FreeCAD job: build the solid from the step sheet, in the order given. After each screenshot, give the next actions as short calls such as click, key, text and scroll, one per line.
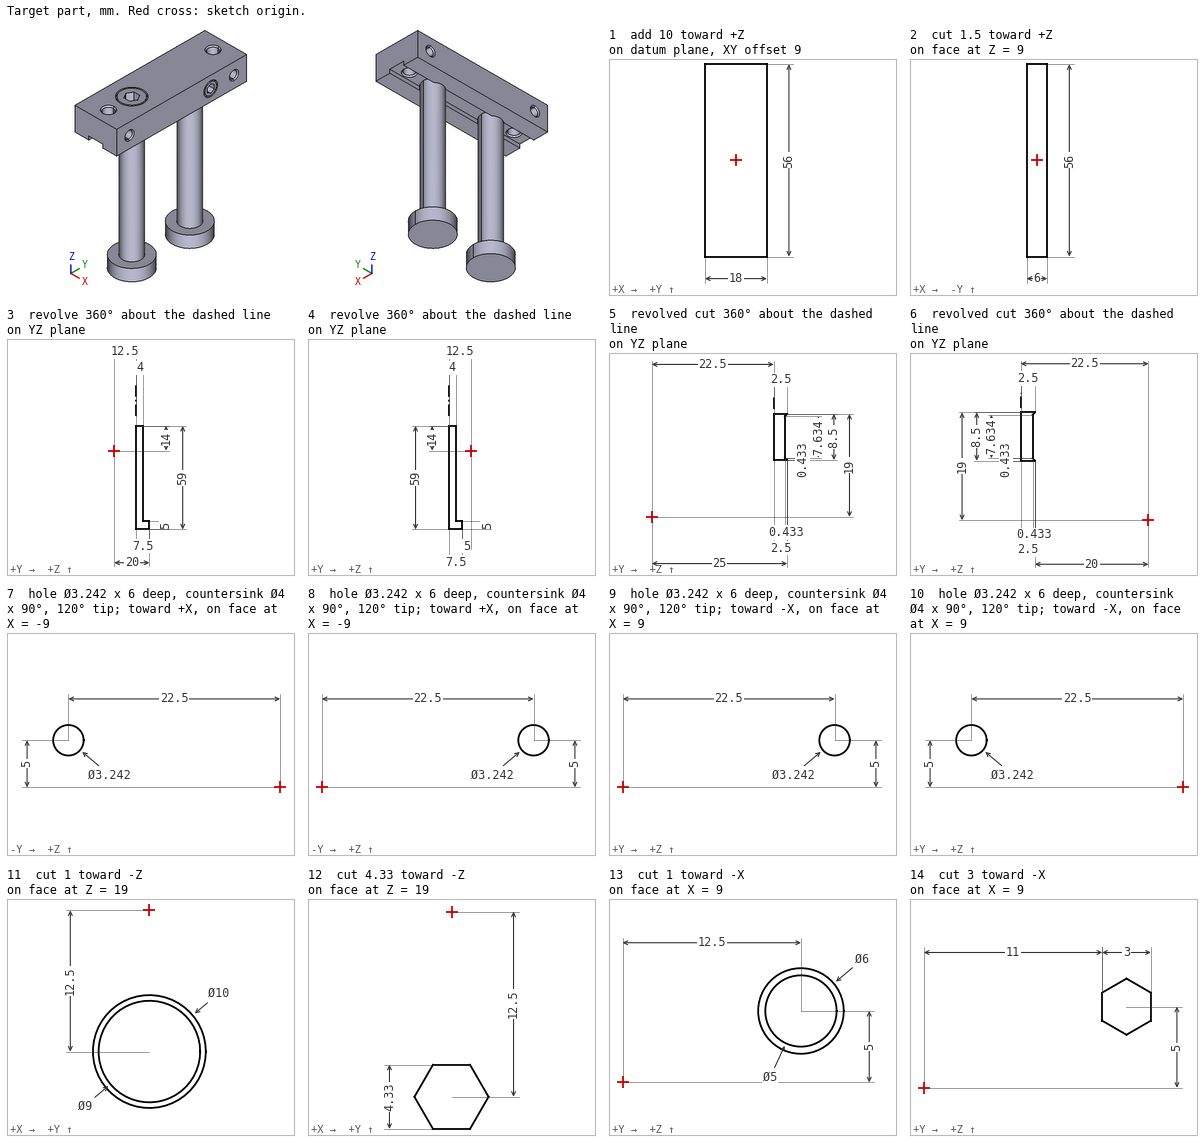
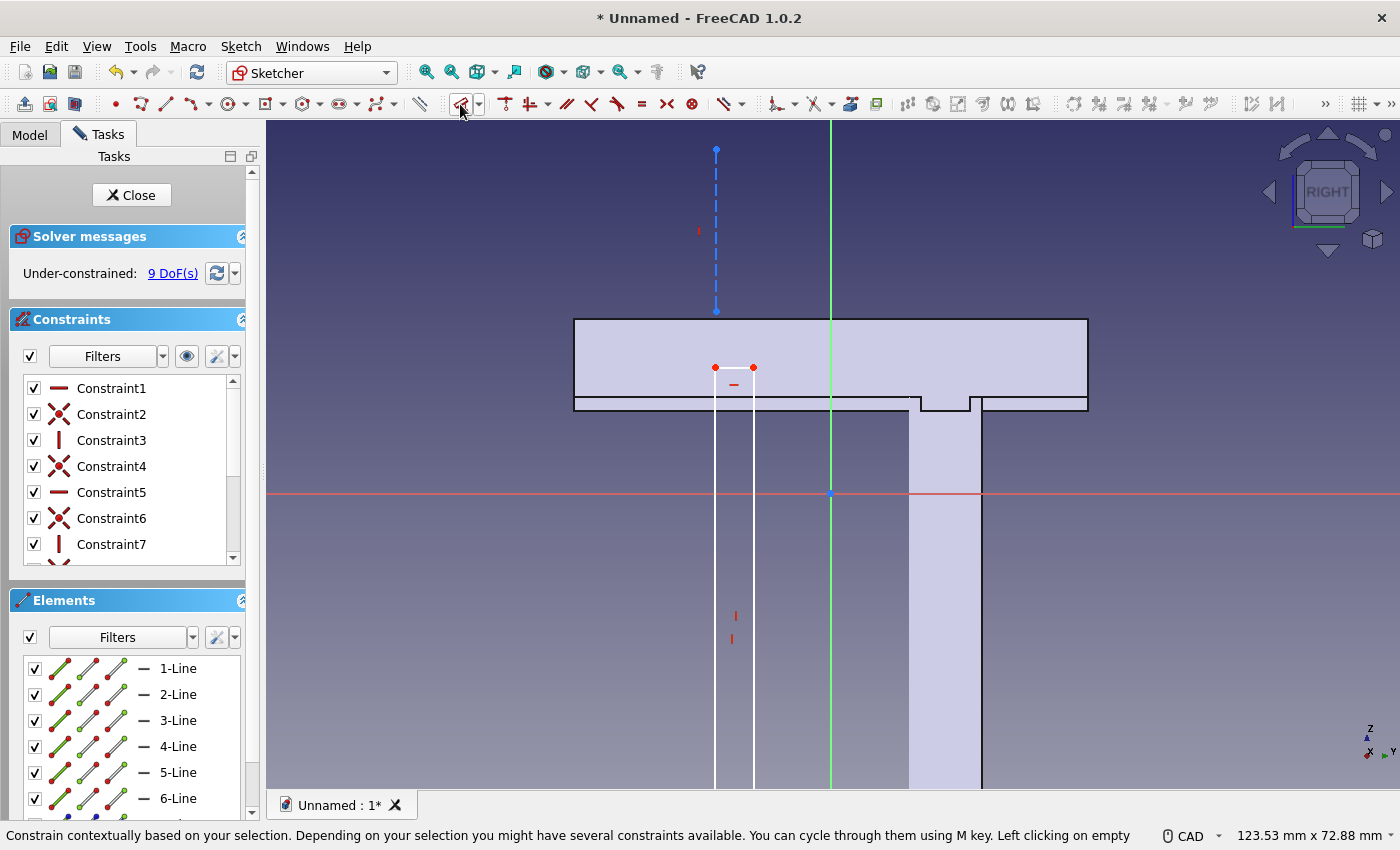
click(742, 368)
click(735, 334)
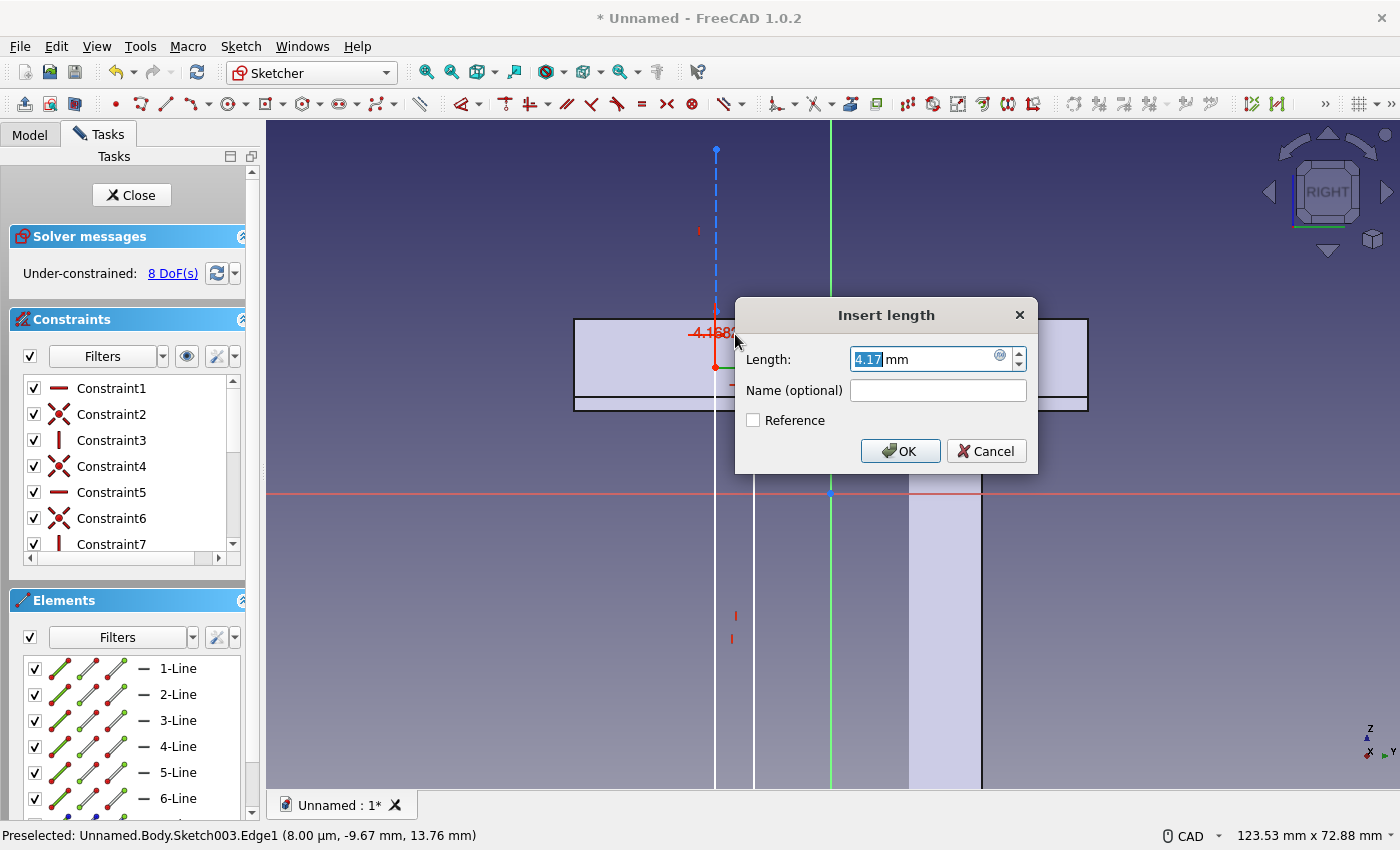
text(4)
key(Return)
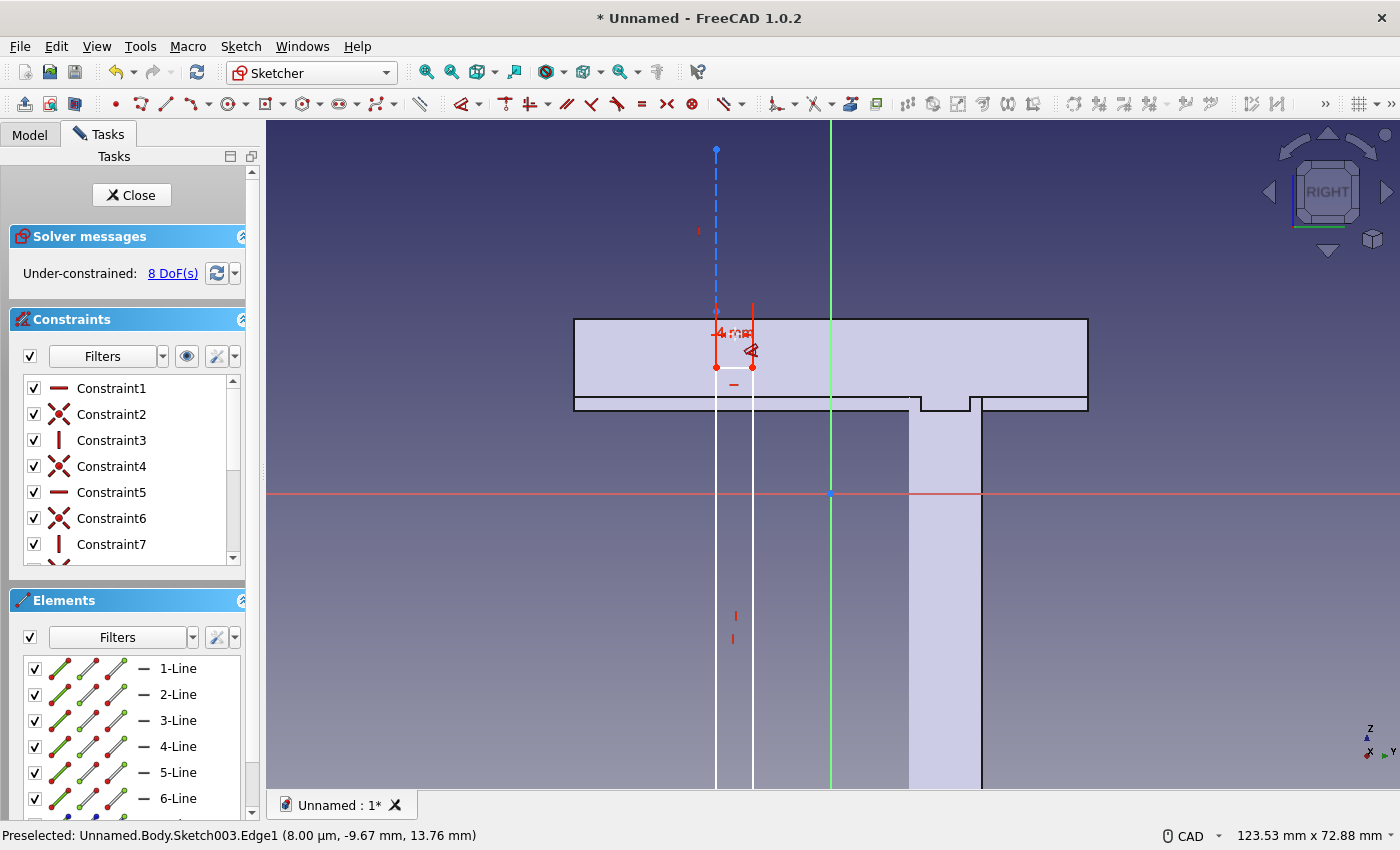
scroll(754, 365, down, 3)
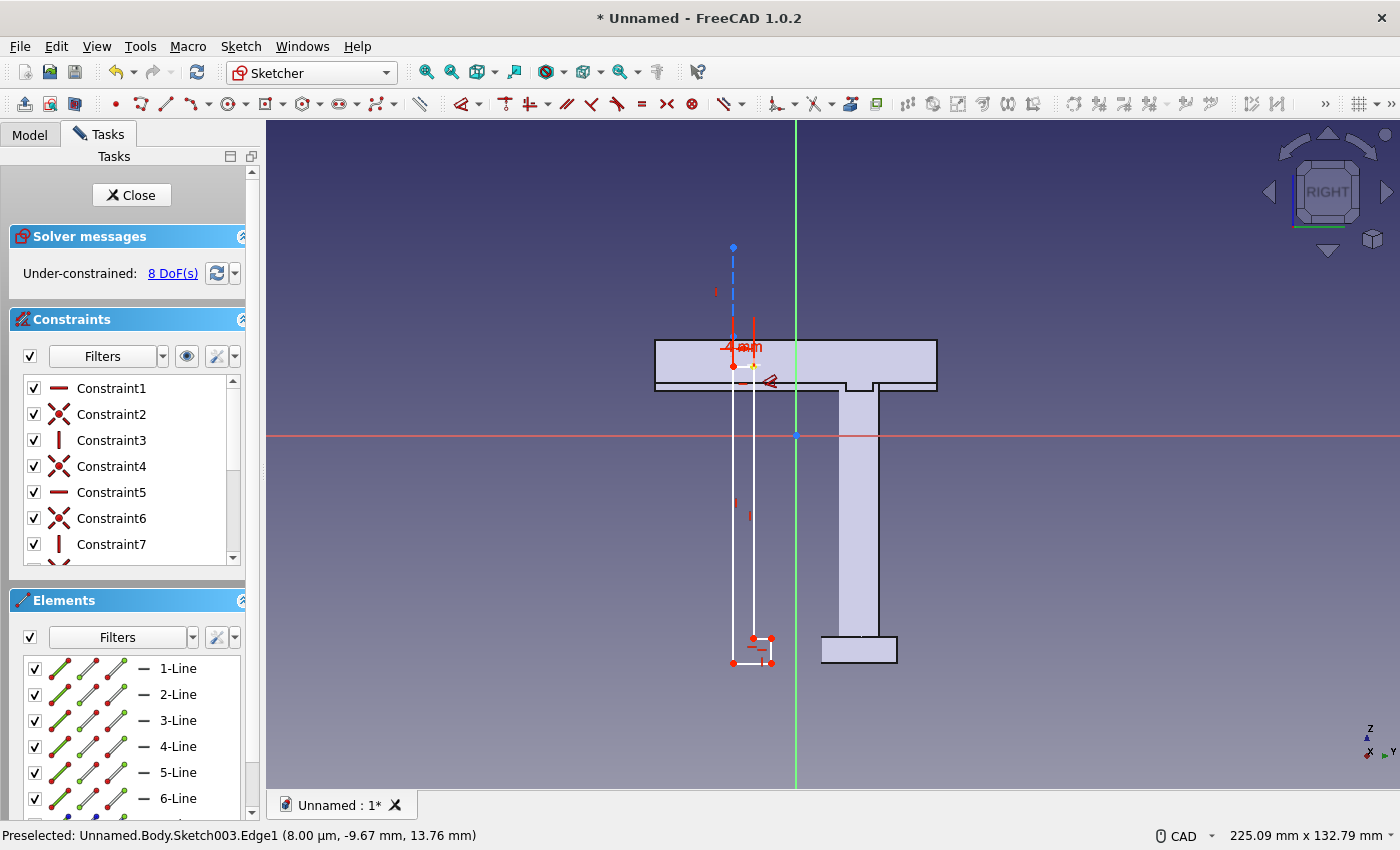
scroll(771, 656, up, 4)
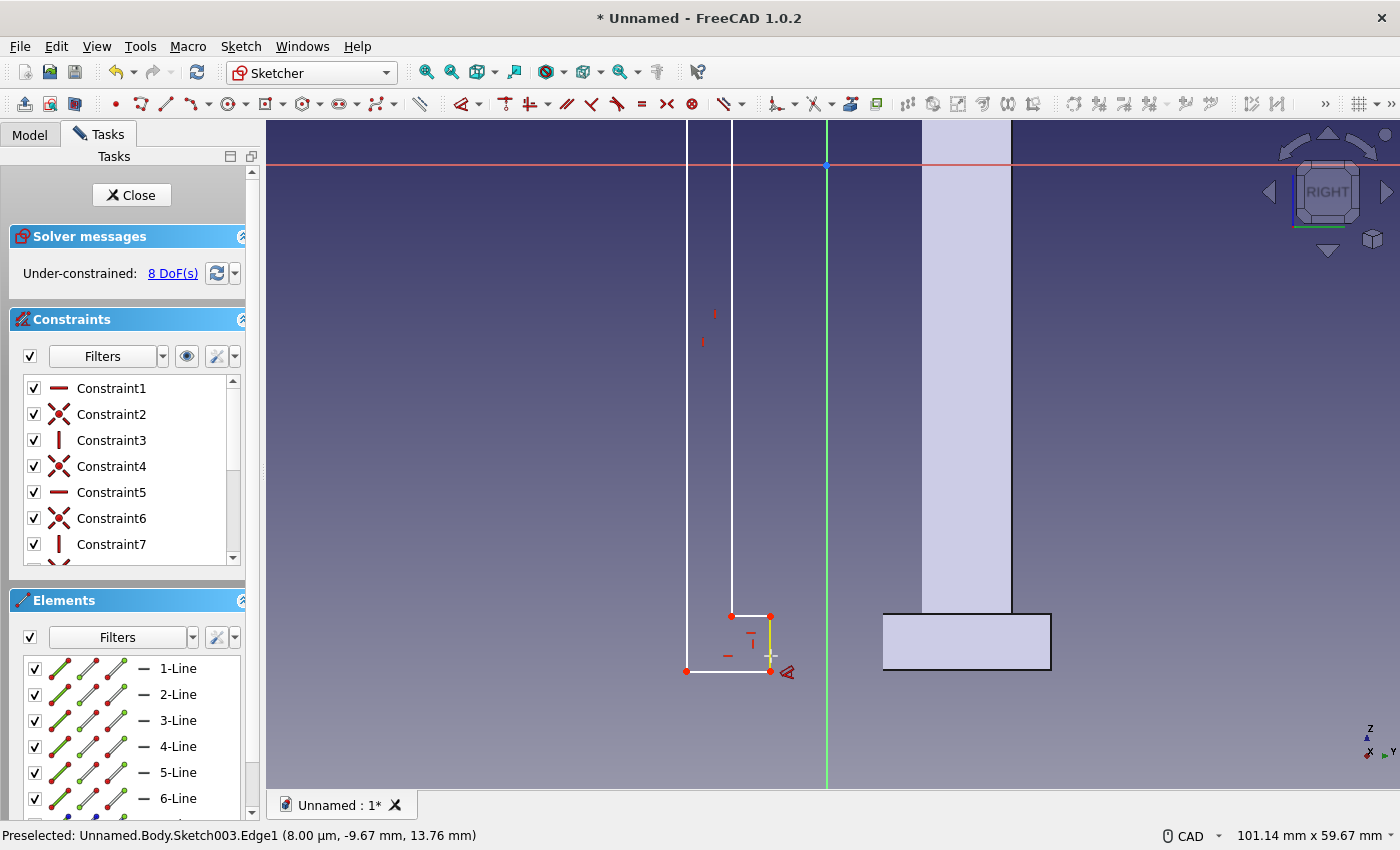
click(770, 655)
click(804, 644)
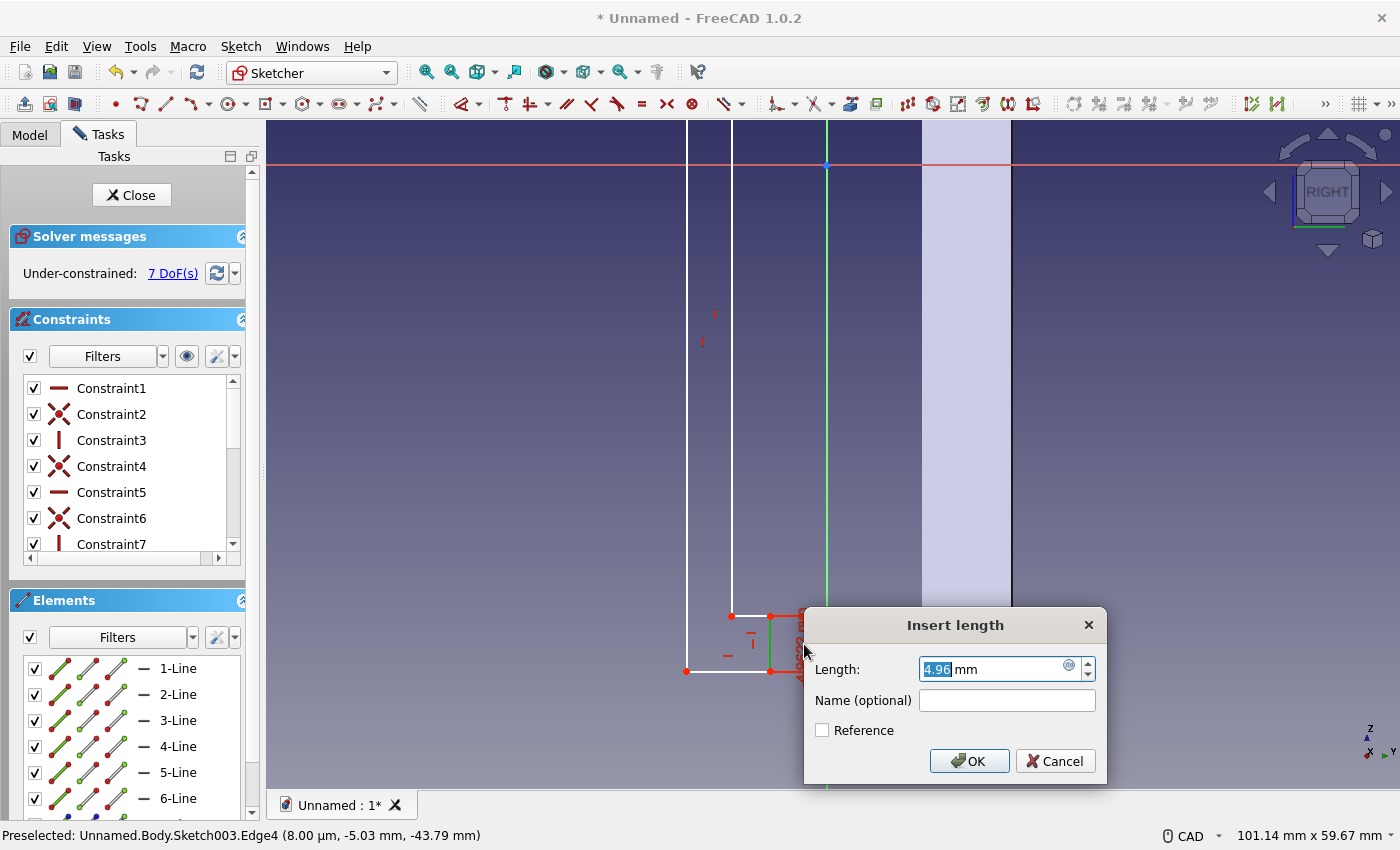
text(5)
key(Return)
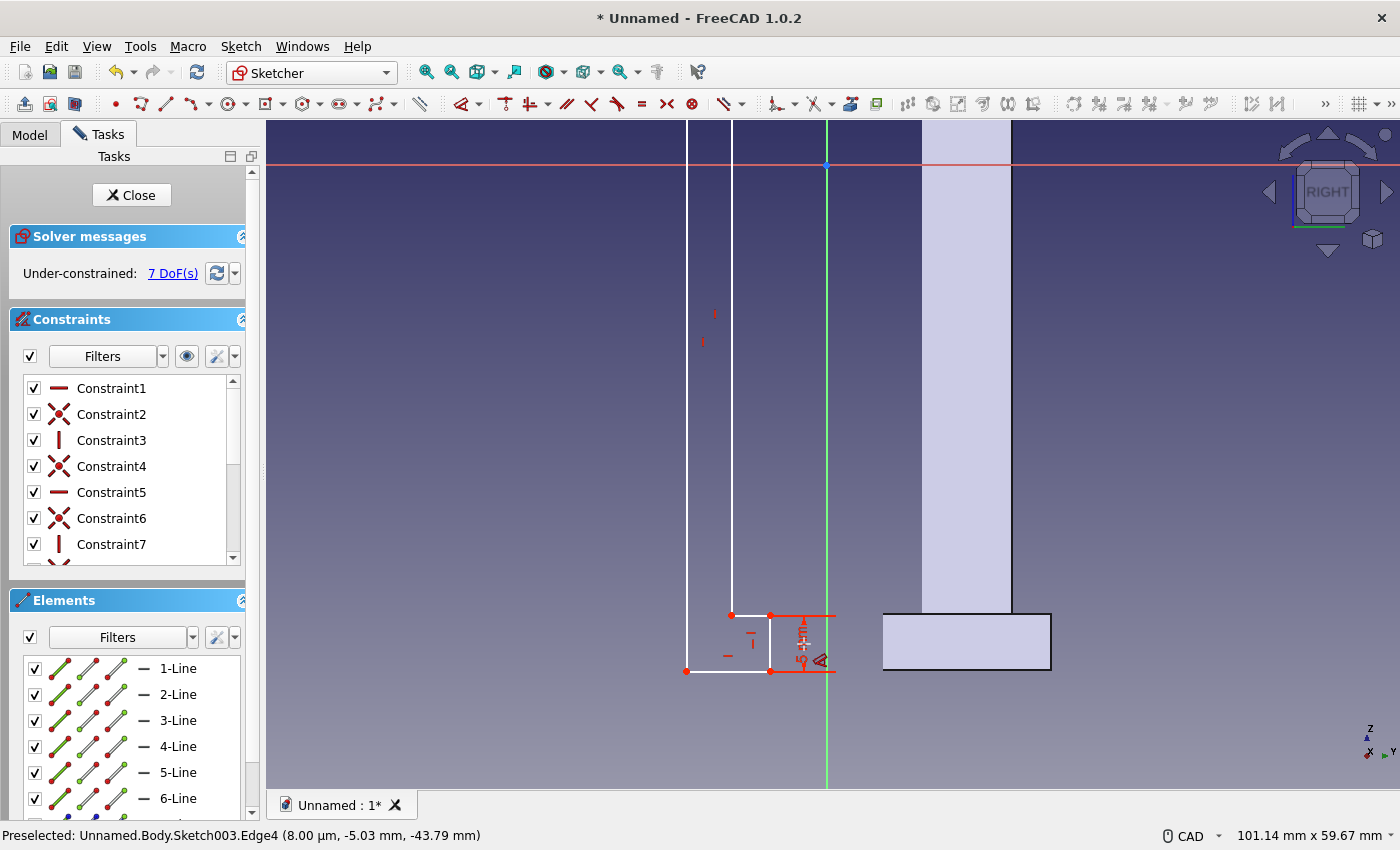
click(687, 209)
click(653, 410)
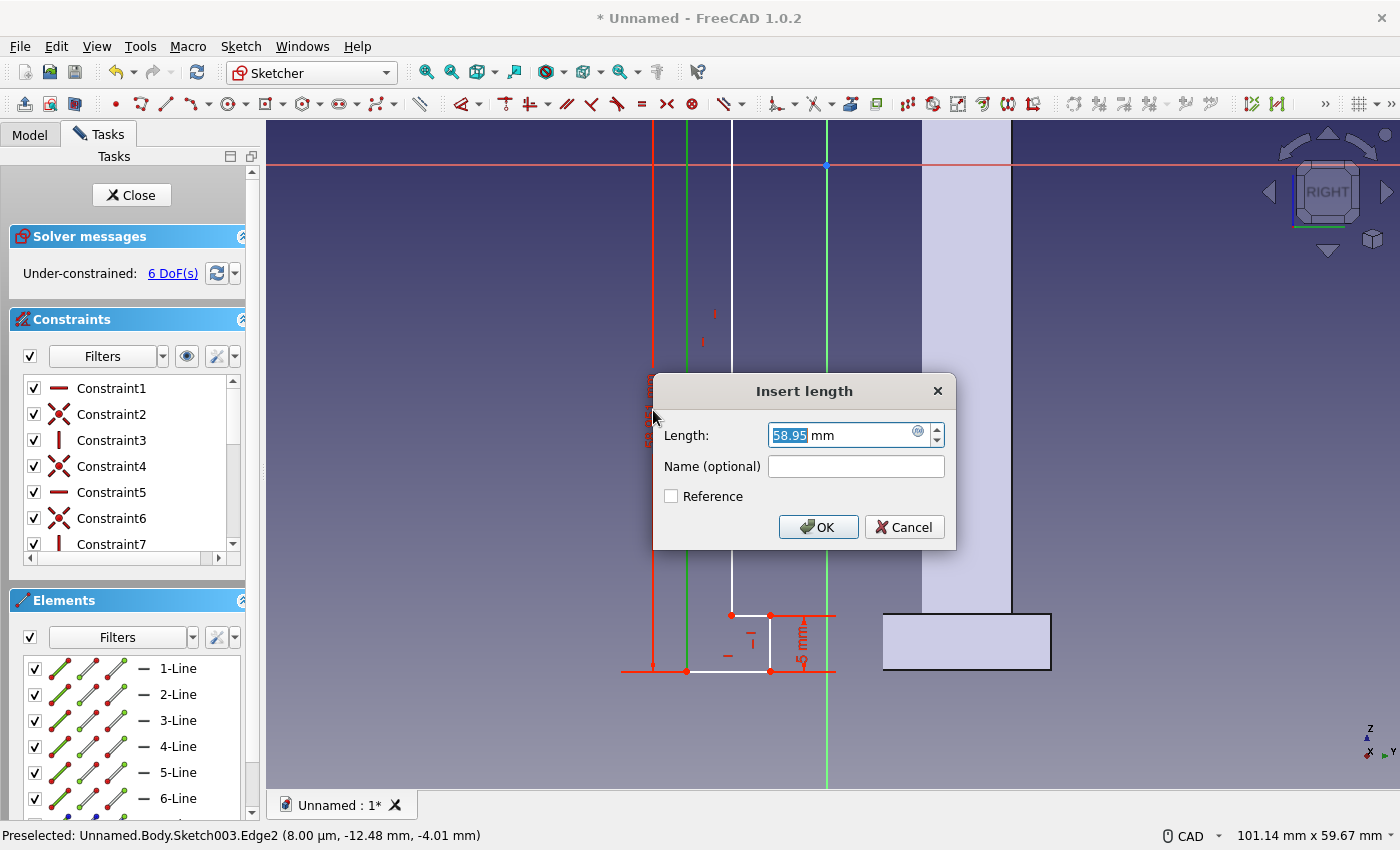
text(59)
key(Return)